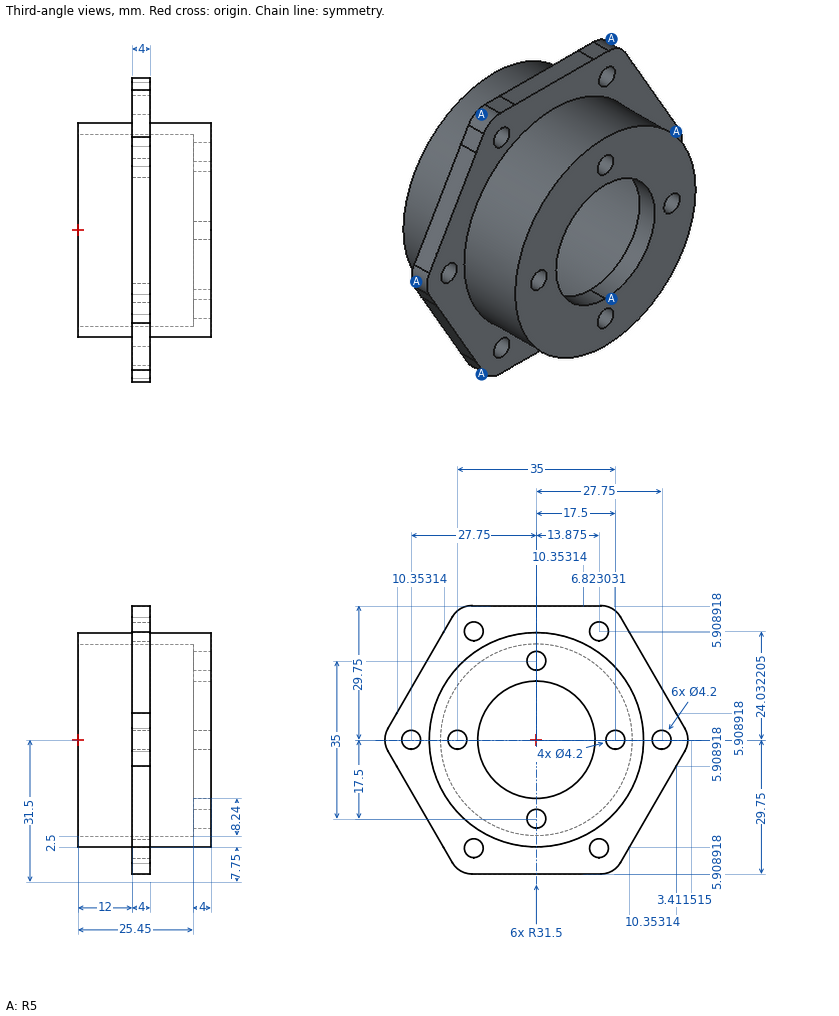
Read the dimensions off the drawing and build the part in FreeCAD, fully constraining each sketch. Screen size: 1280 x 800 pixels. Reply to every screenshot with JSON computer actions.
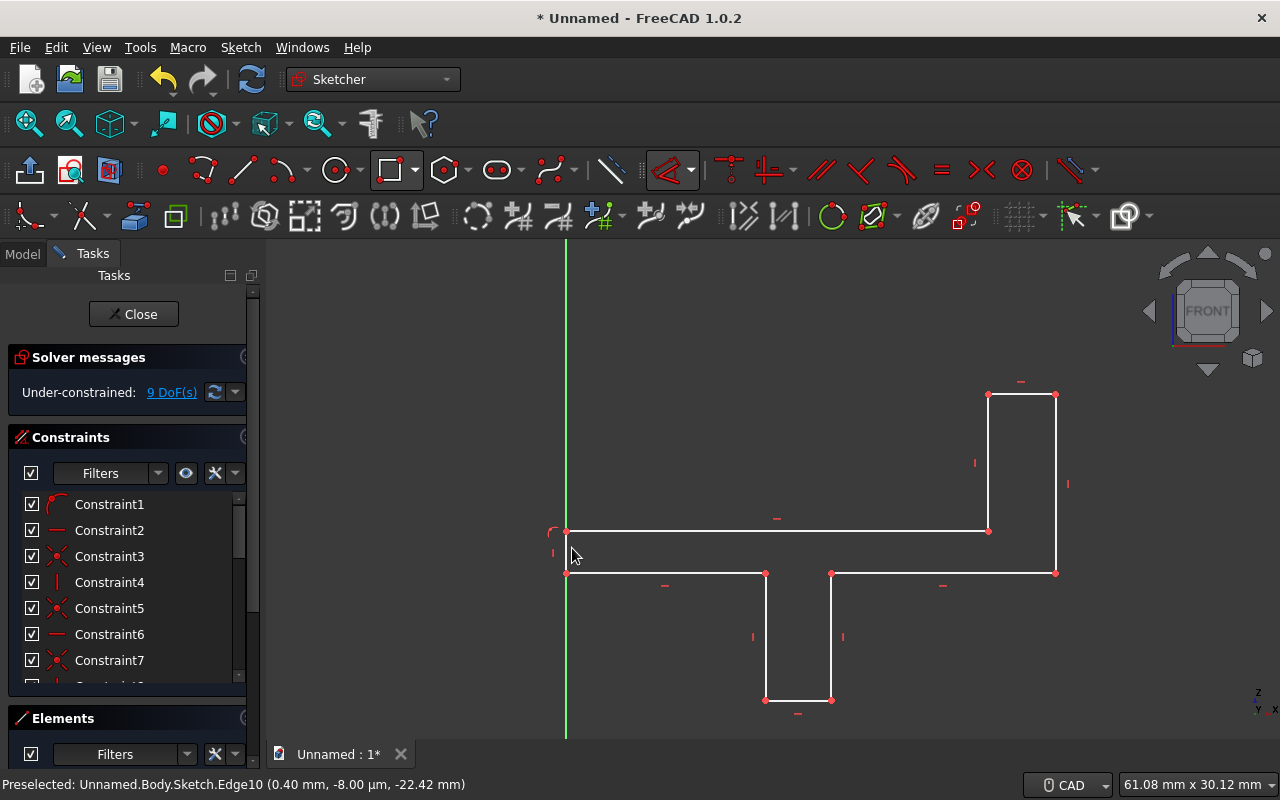
{"action": "left_click", "coordinate": [666, 170]}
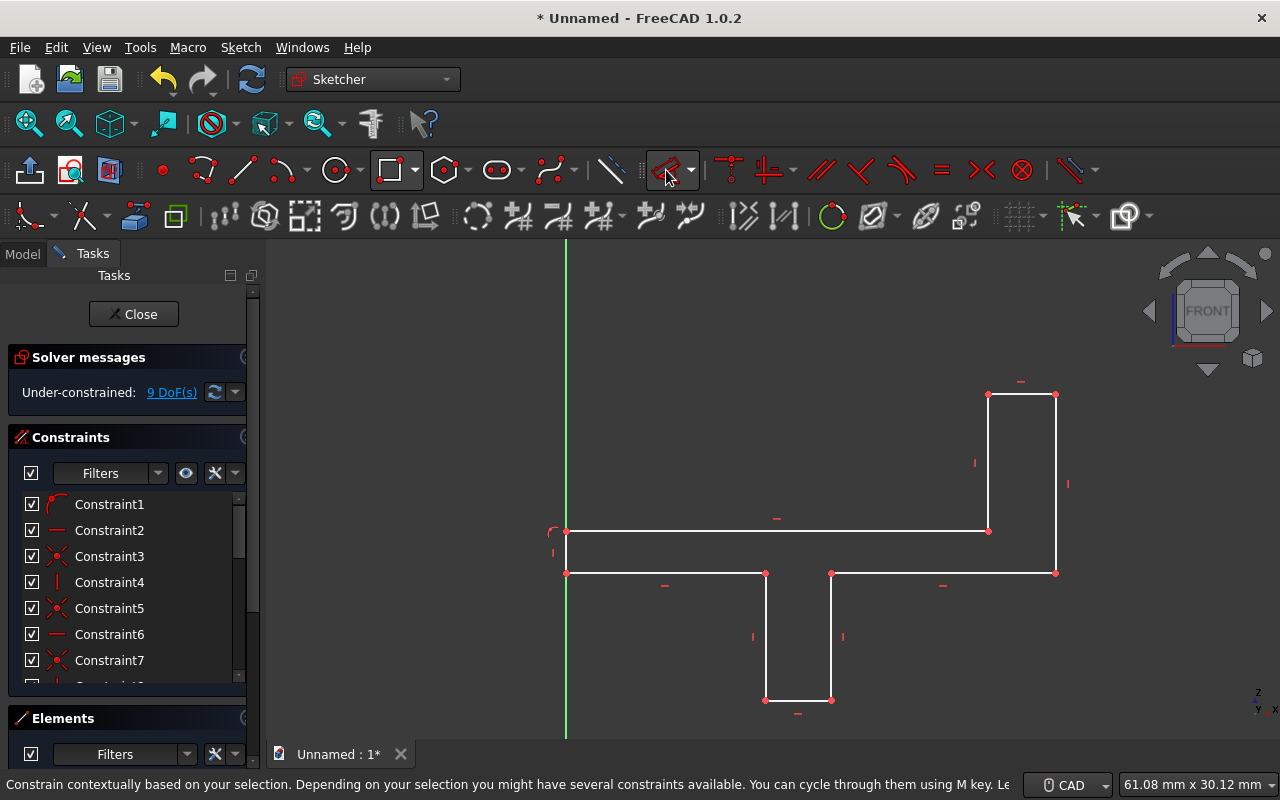
{"action": "left_click", "coordinate": [1008, 394]}
{"action": "left_click", "coordinate": [1022, 360]}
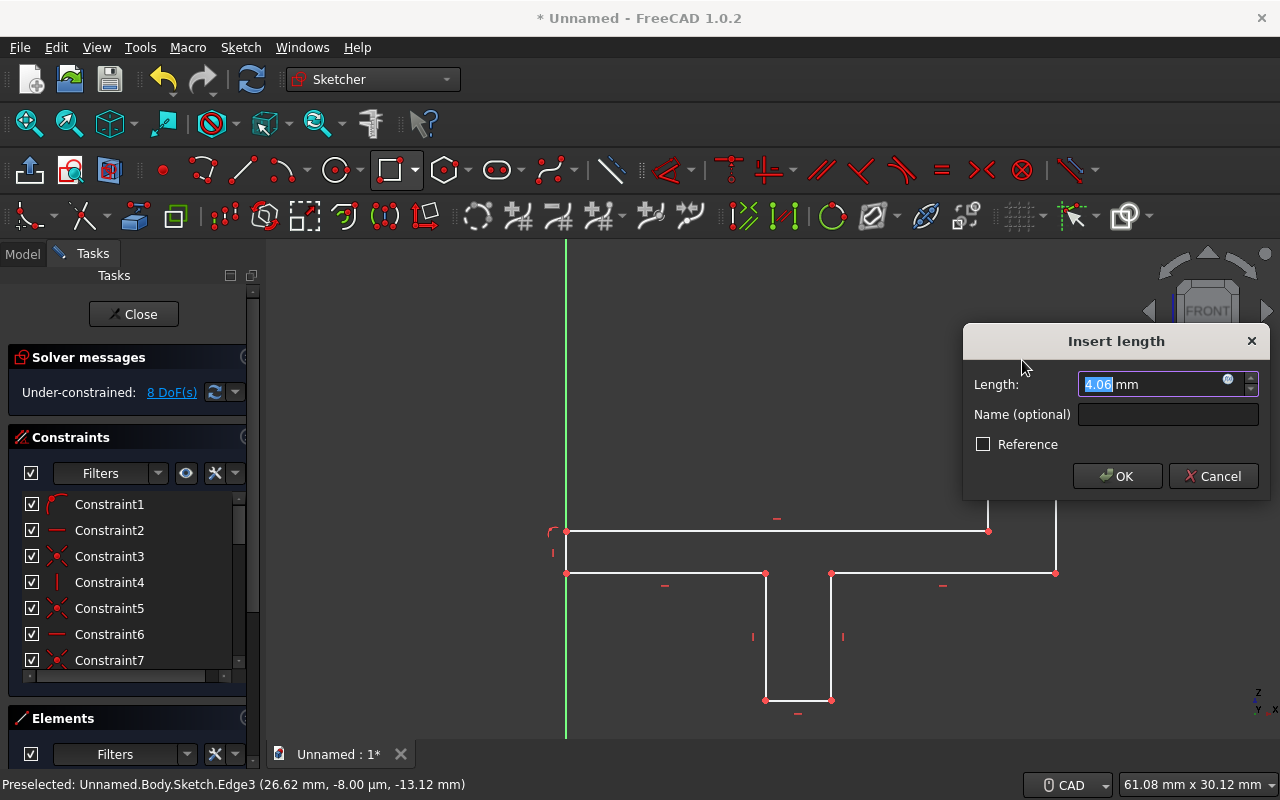
{"action": "type", "text": "4"}
{"action": "key", "text": "Return"}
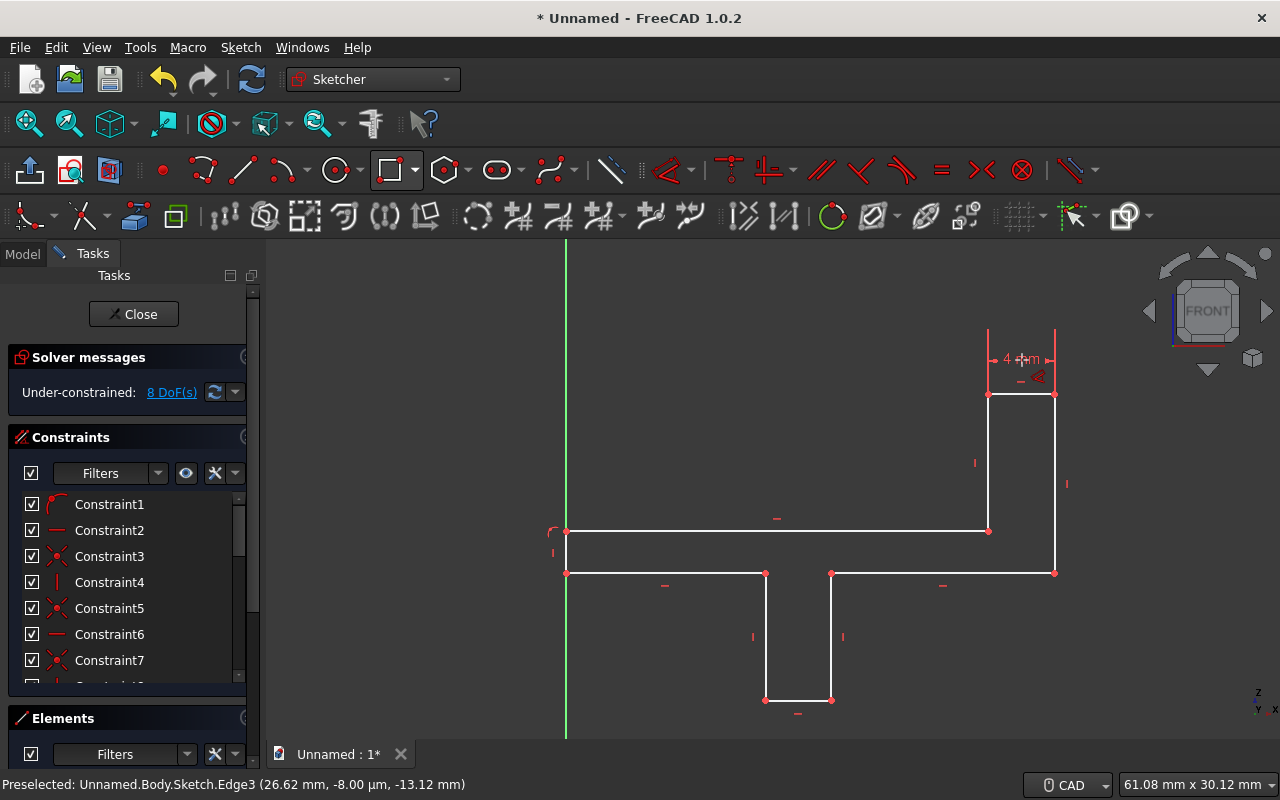
{"action": "left_click", "coordinate": [812, 701]}
{"action": "left_click", "coordinate": [799, 667]}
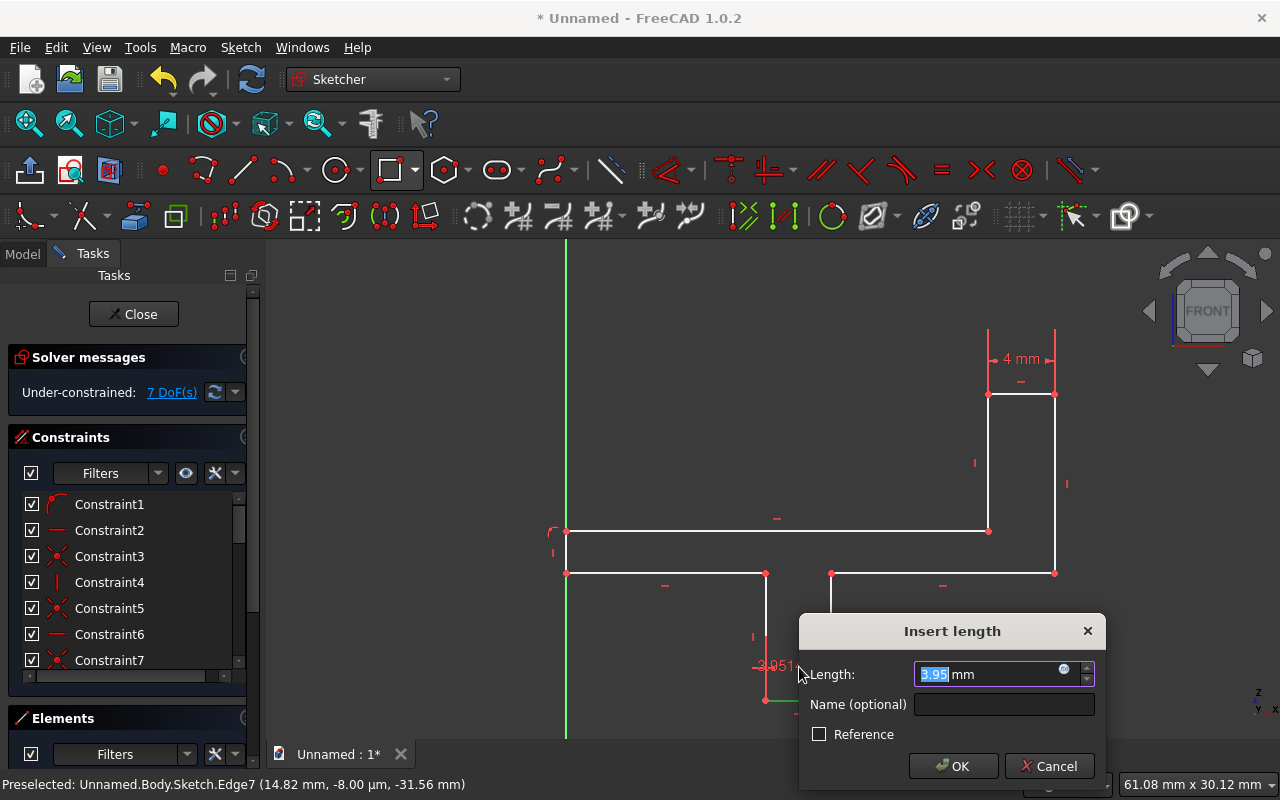
{"action": "type", "text": "4"}
{"action": "key", "text": "Return"}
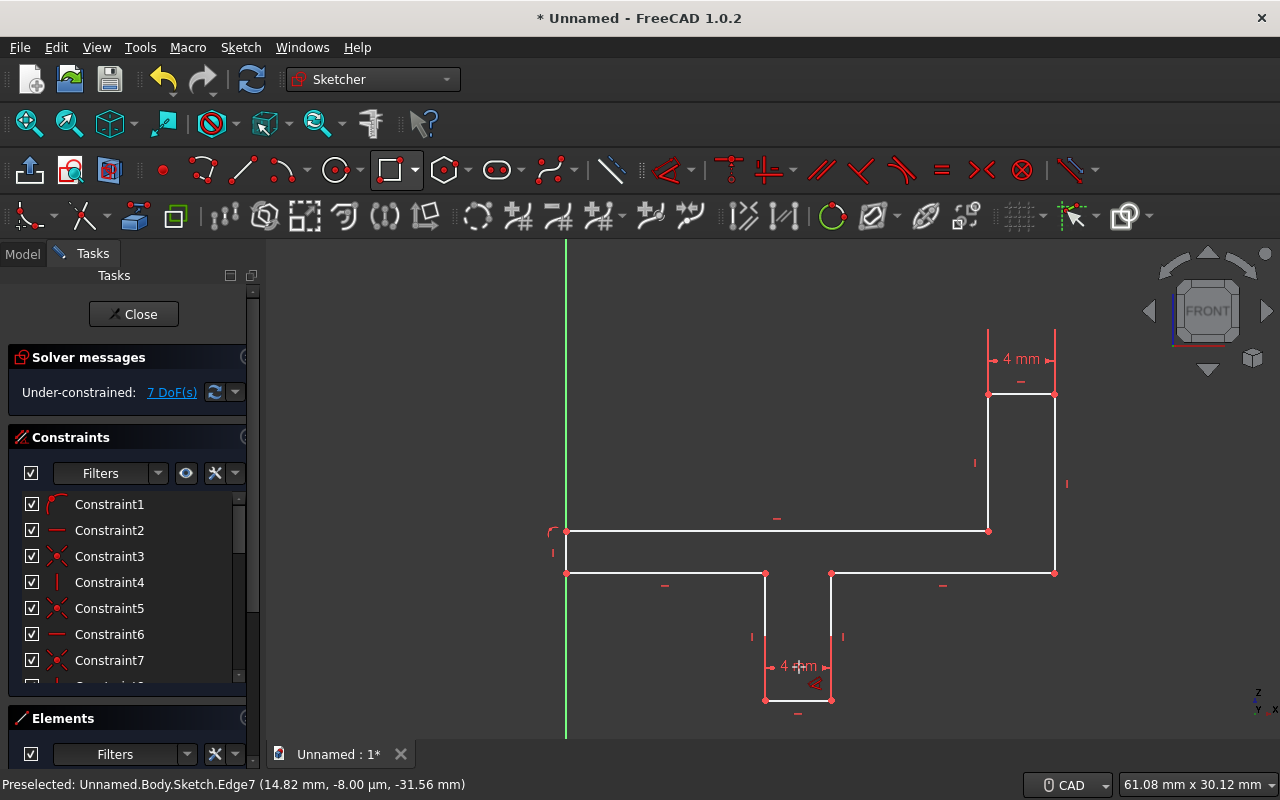
{"action": "left_click", "coordinate": [705, 573]}
{"action": "left_click", "coordinate": [666, 607]}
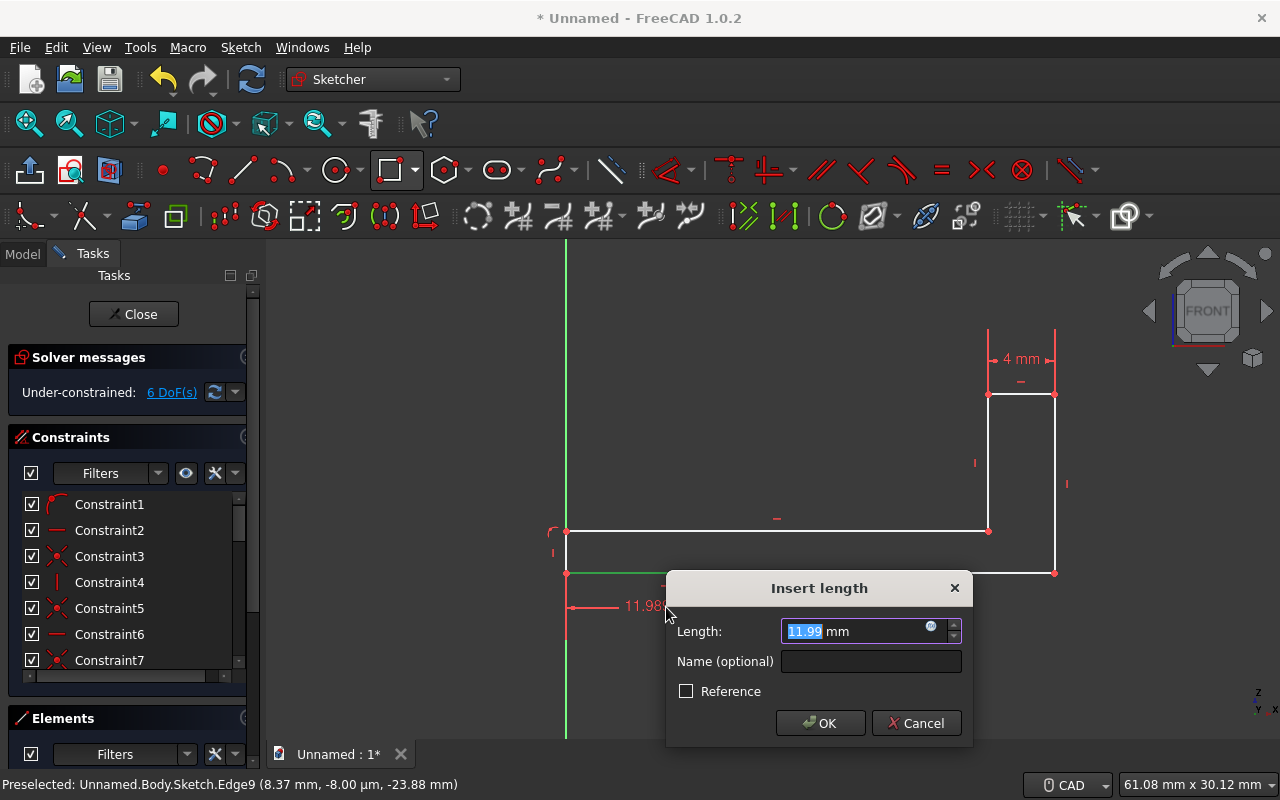
{"action": "type", "text": "12"}
{"action": "key", "text": "Return"}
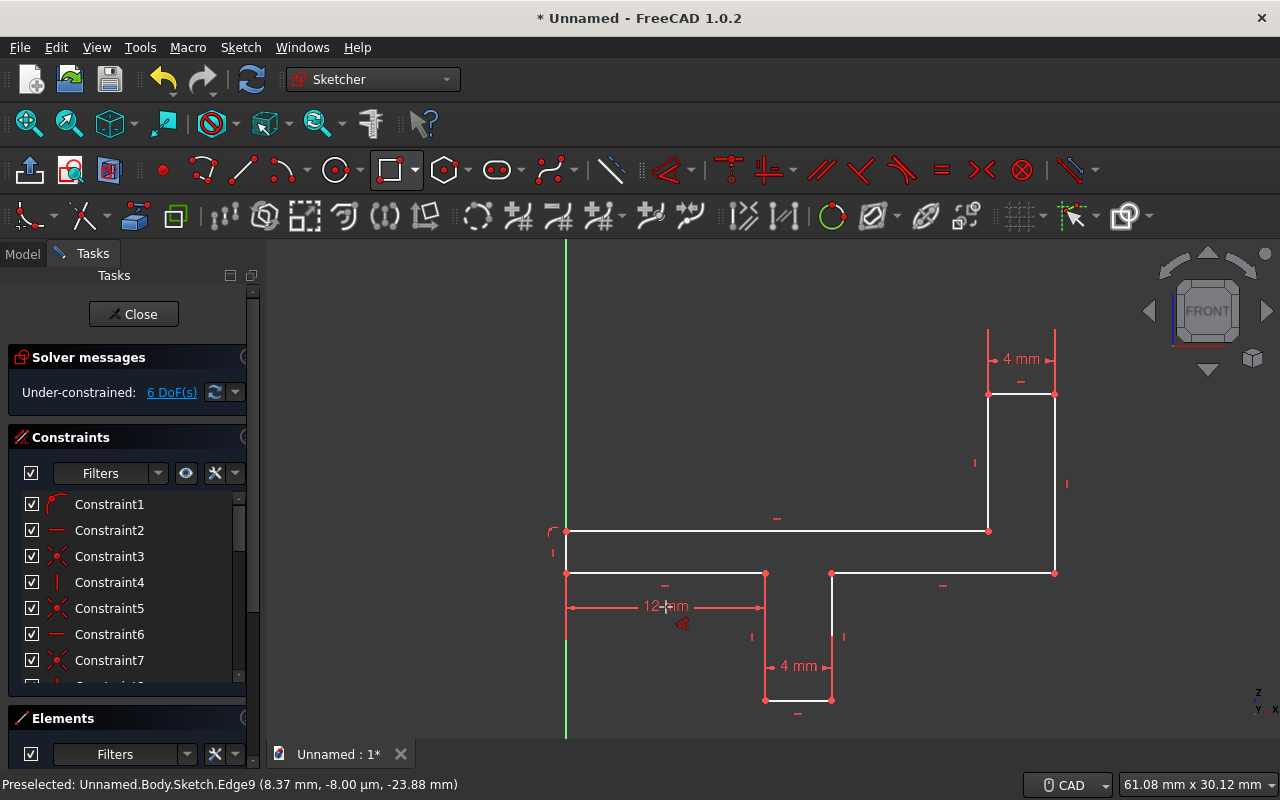
{"action": "left_click", "coordinate": [566, 560]}
{"action": "left_click", "coordinate": [532, 552]}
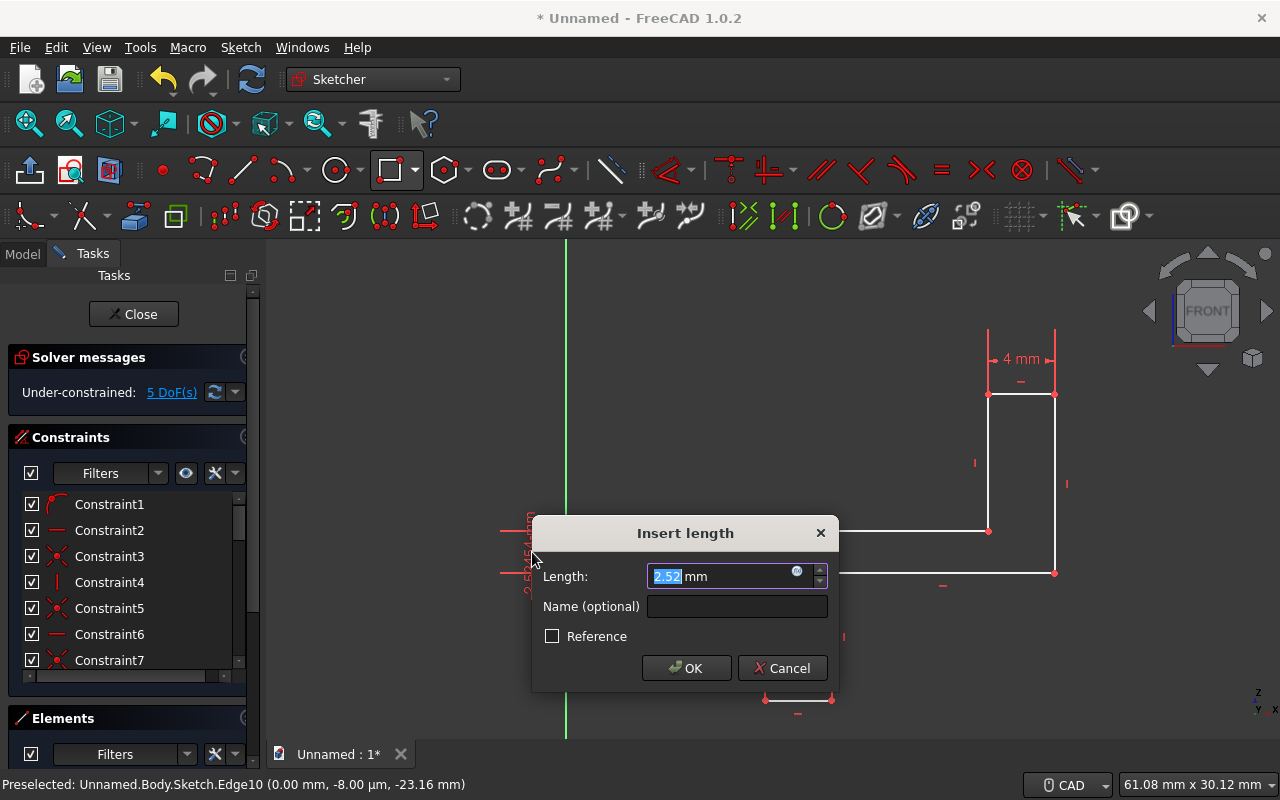
{"action": "type", "text": "2.5"}
{"action": "key", "text": "Return"}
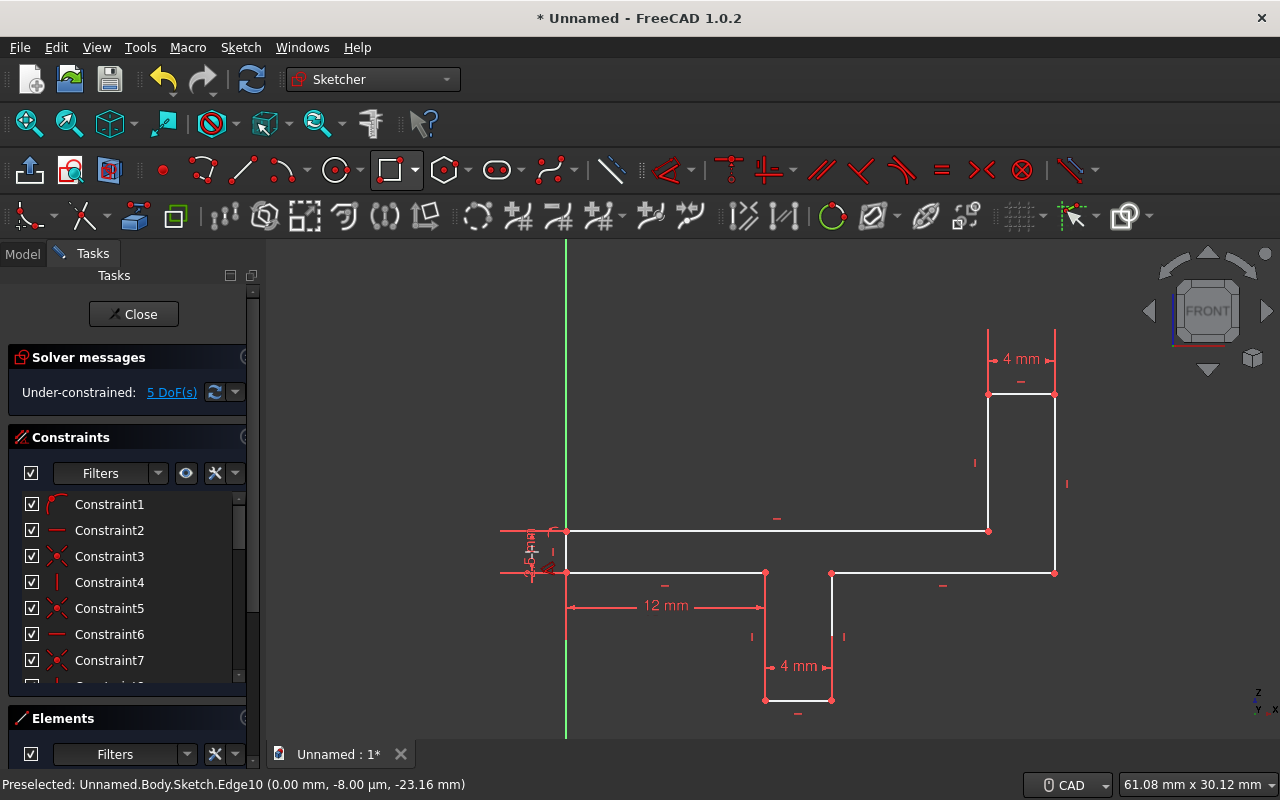
{"action": "left_click", "coordinate": [988, 490]}
{"action": "left_click", "coordinate": [1022, 463]}